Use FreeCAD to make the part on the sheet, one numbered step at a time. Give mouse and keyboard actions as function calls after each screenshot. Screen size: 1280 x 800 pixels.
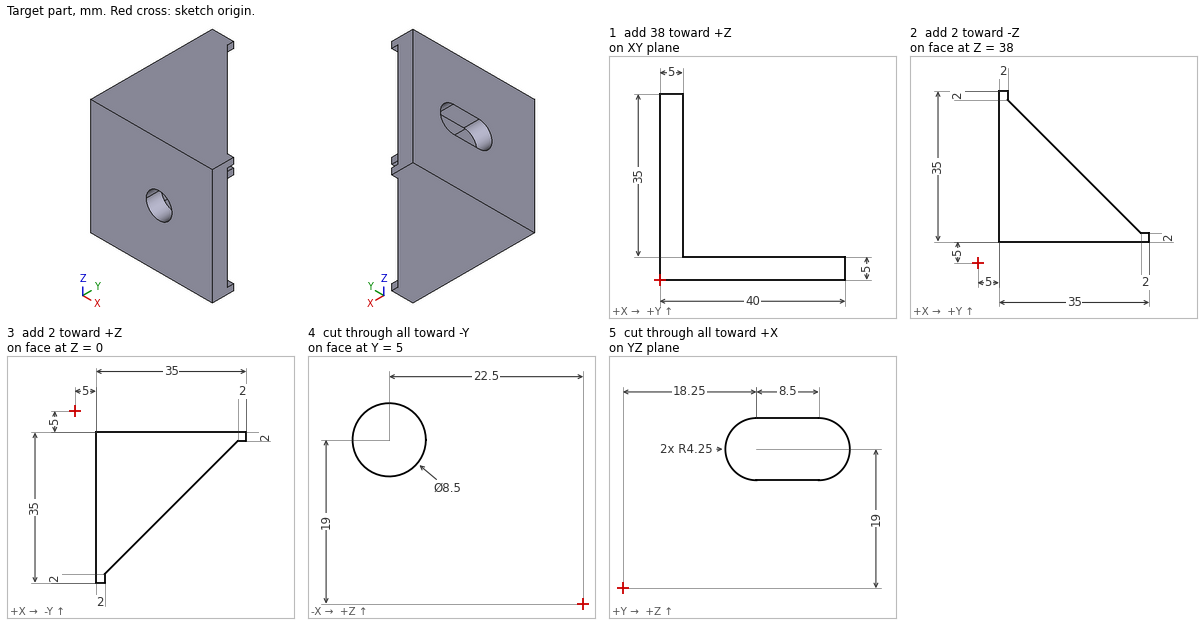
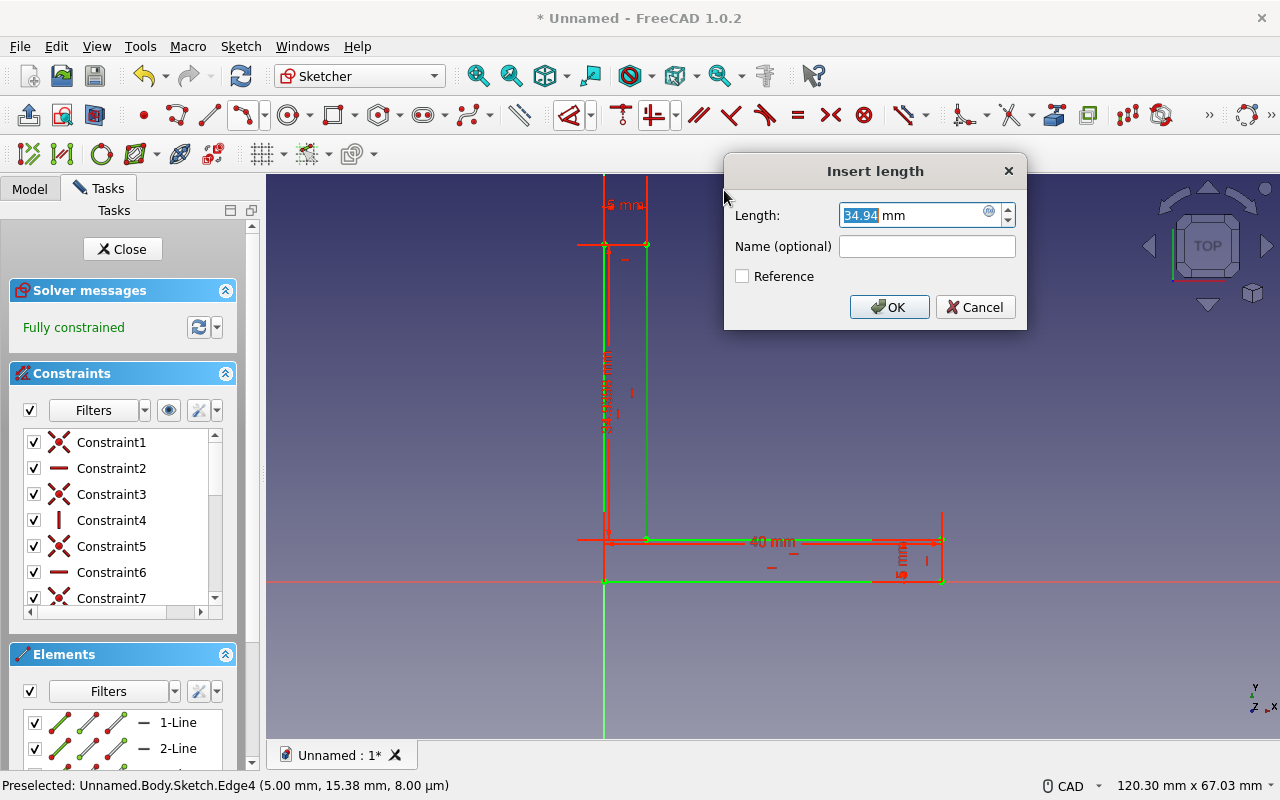
text(35)
key(Return)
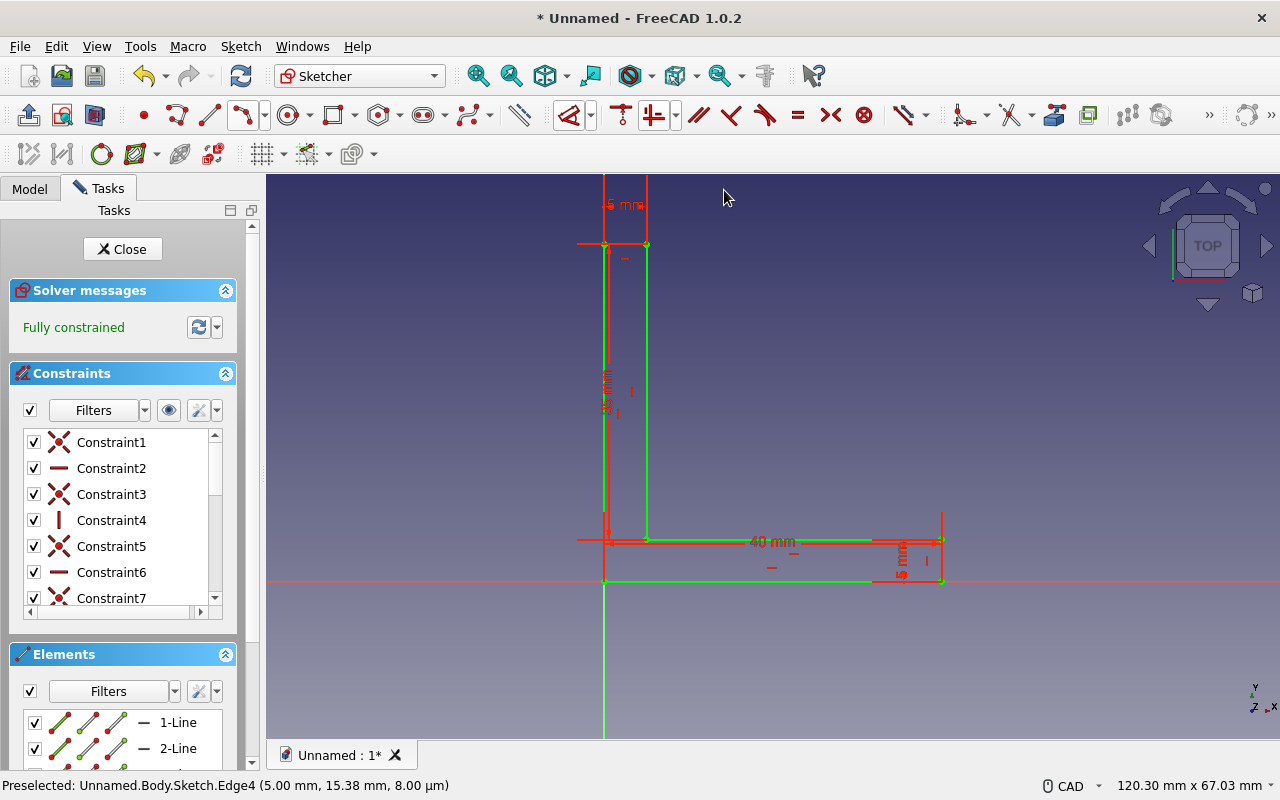
click(123, 249)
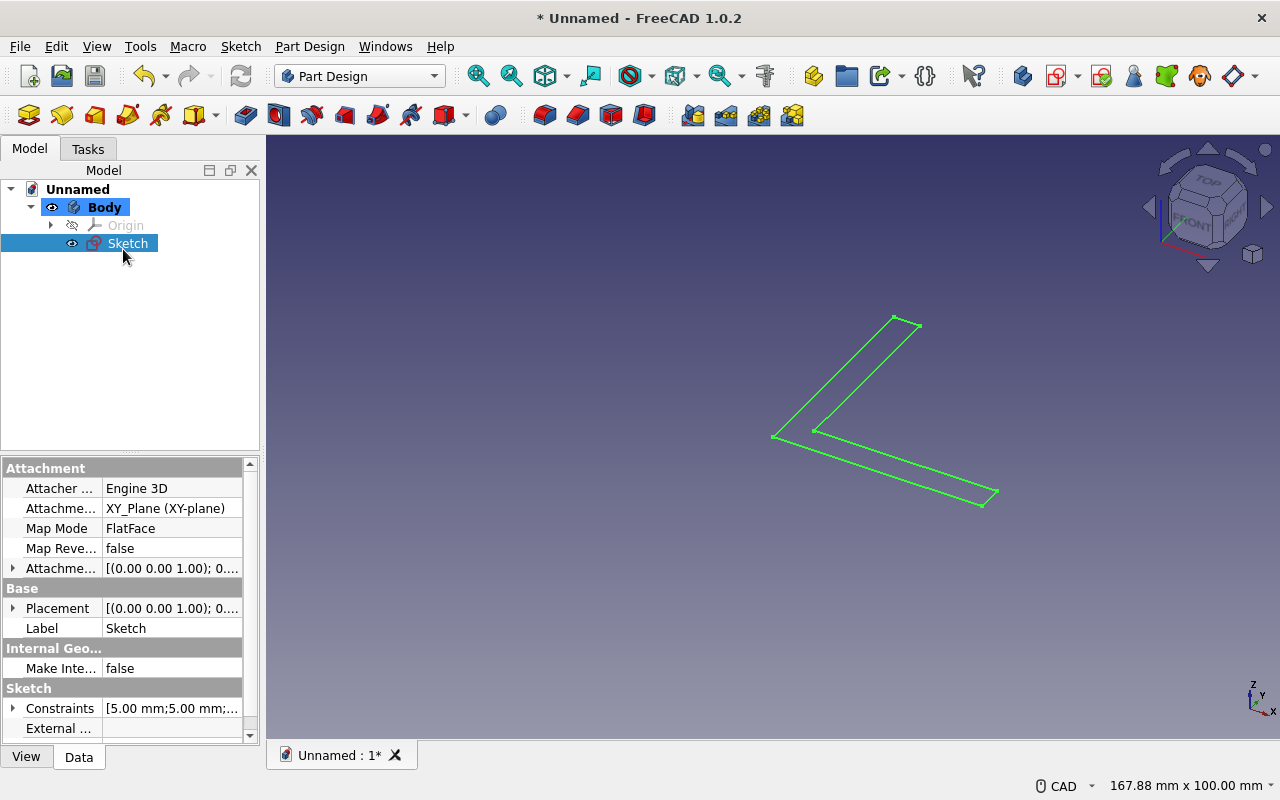
click(29, 116)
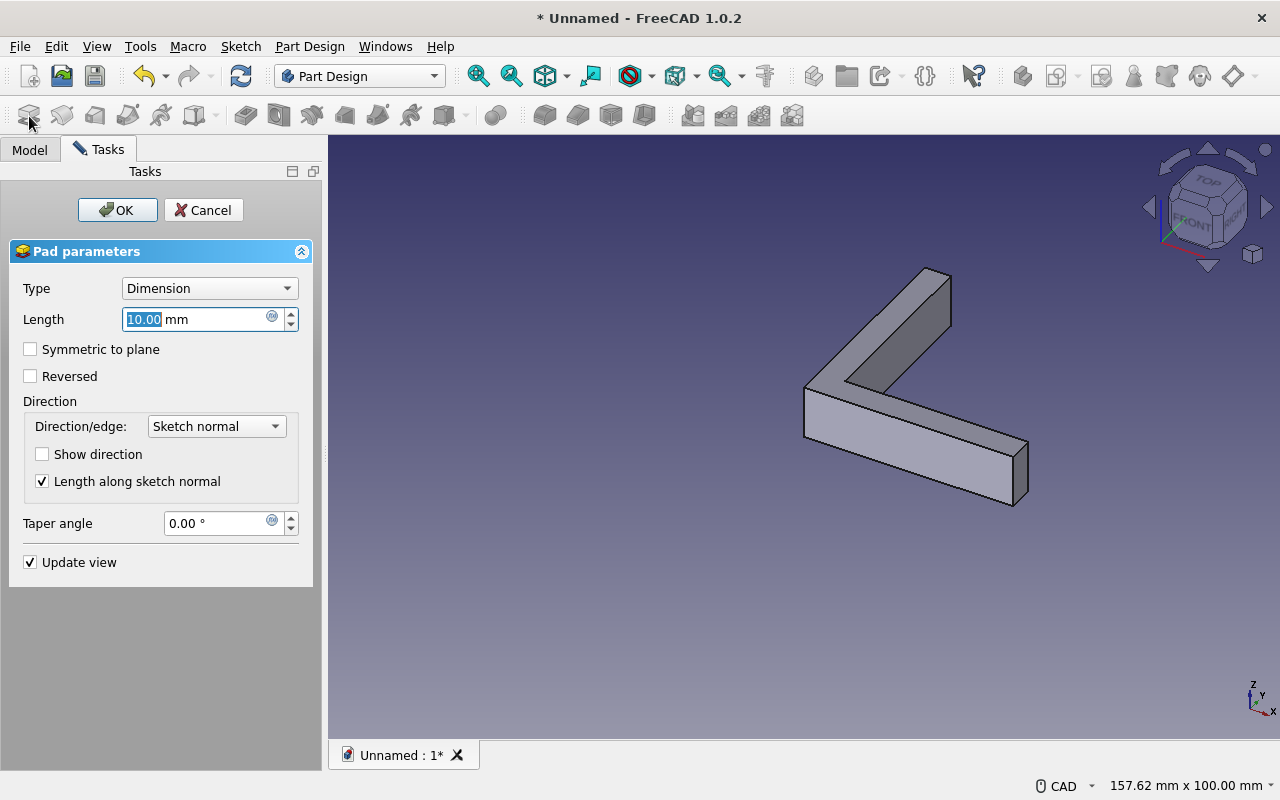
text(38)
key(Tab)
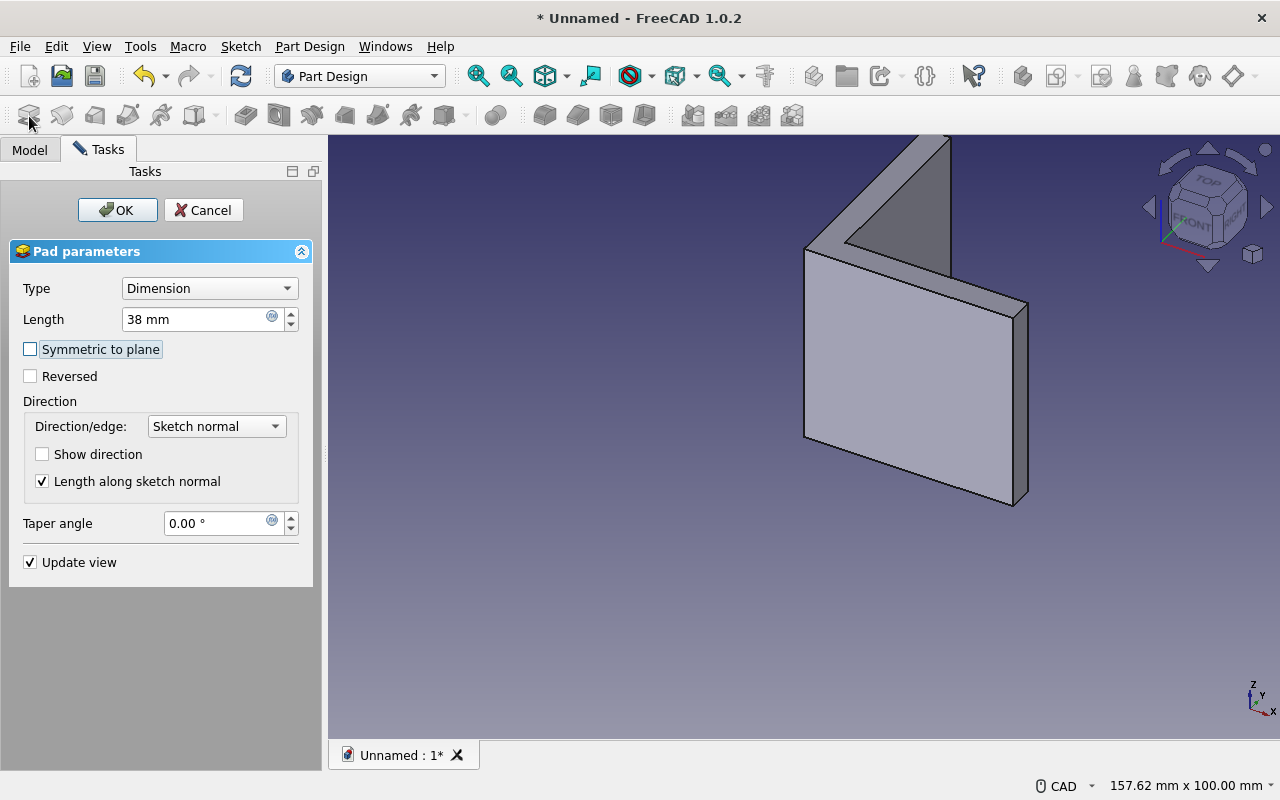
click(118, 210)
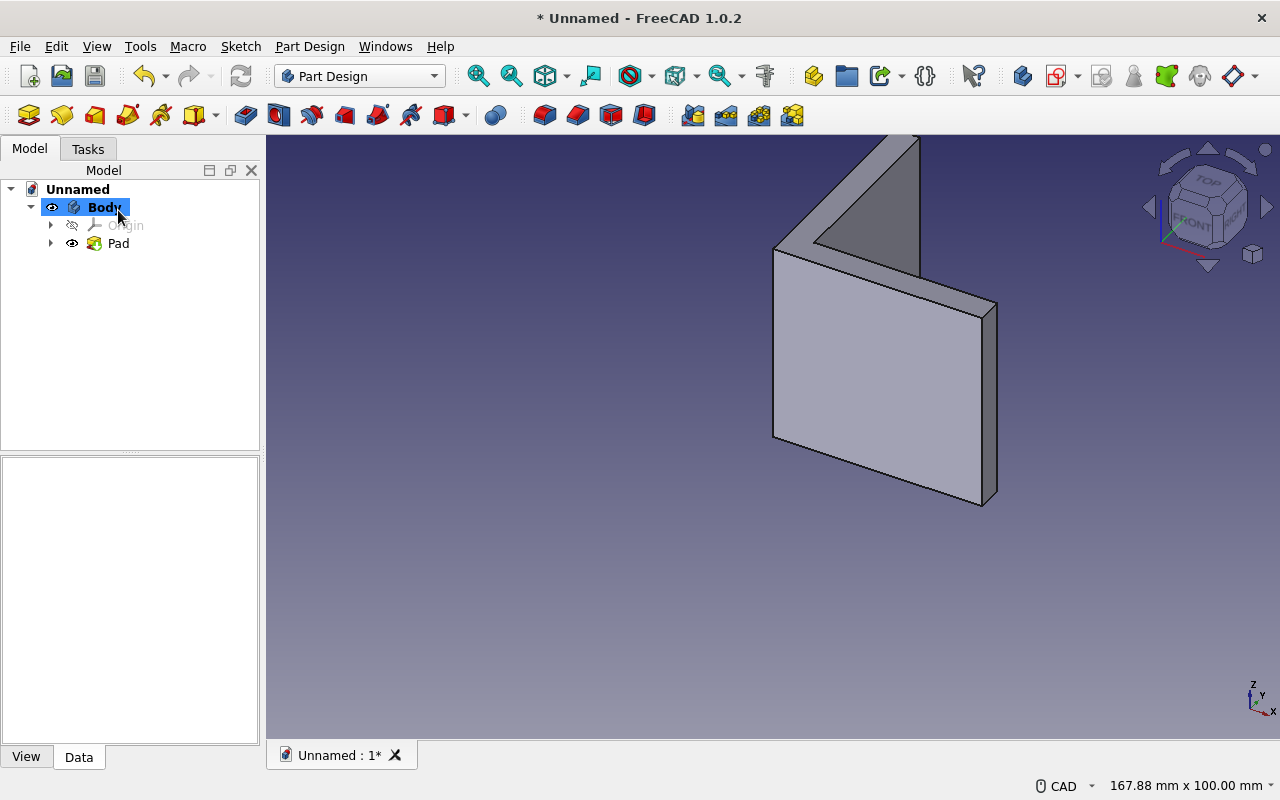
click(479, 76)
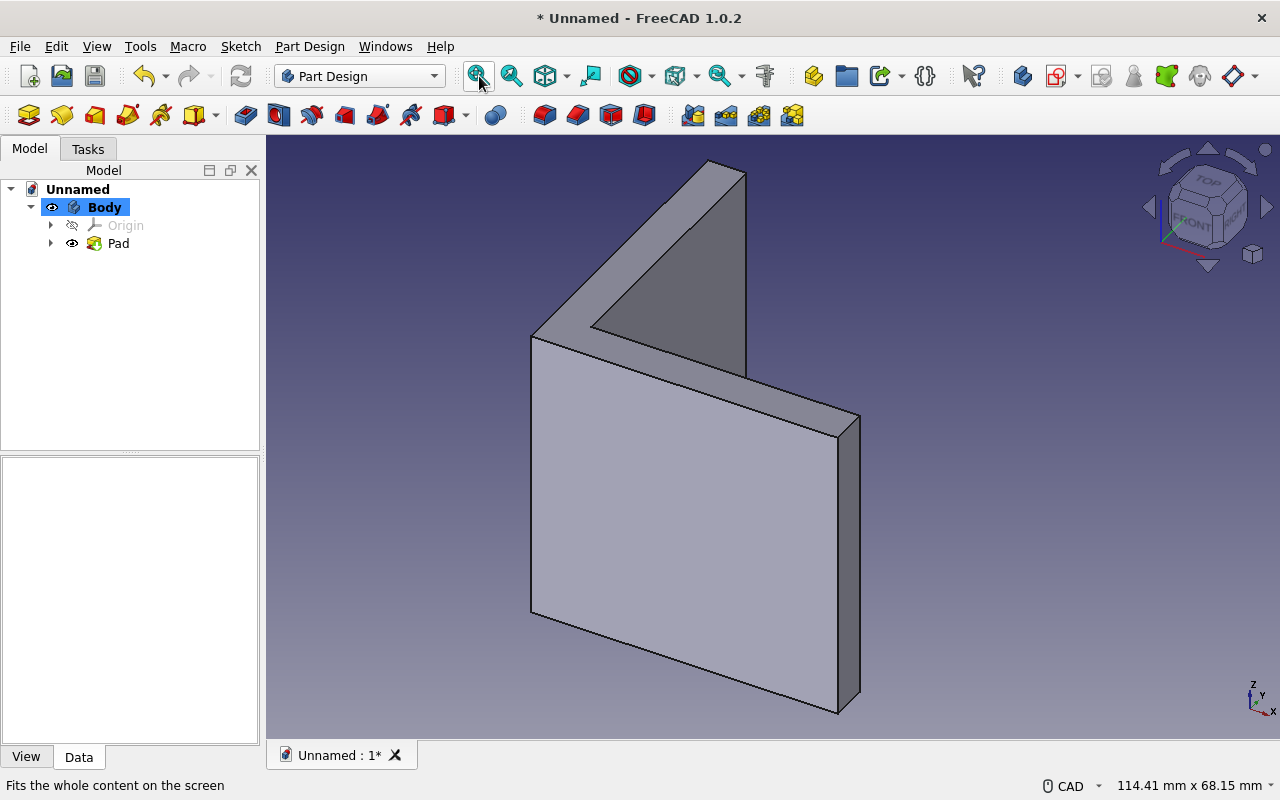
click(565, 330)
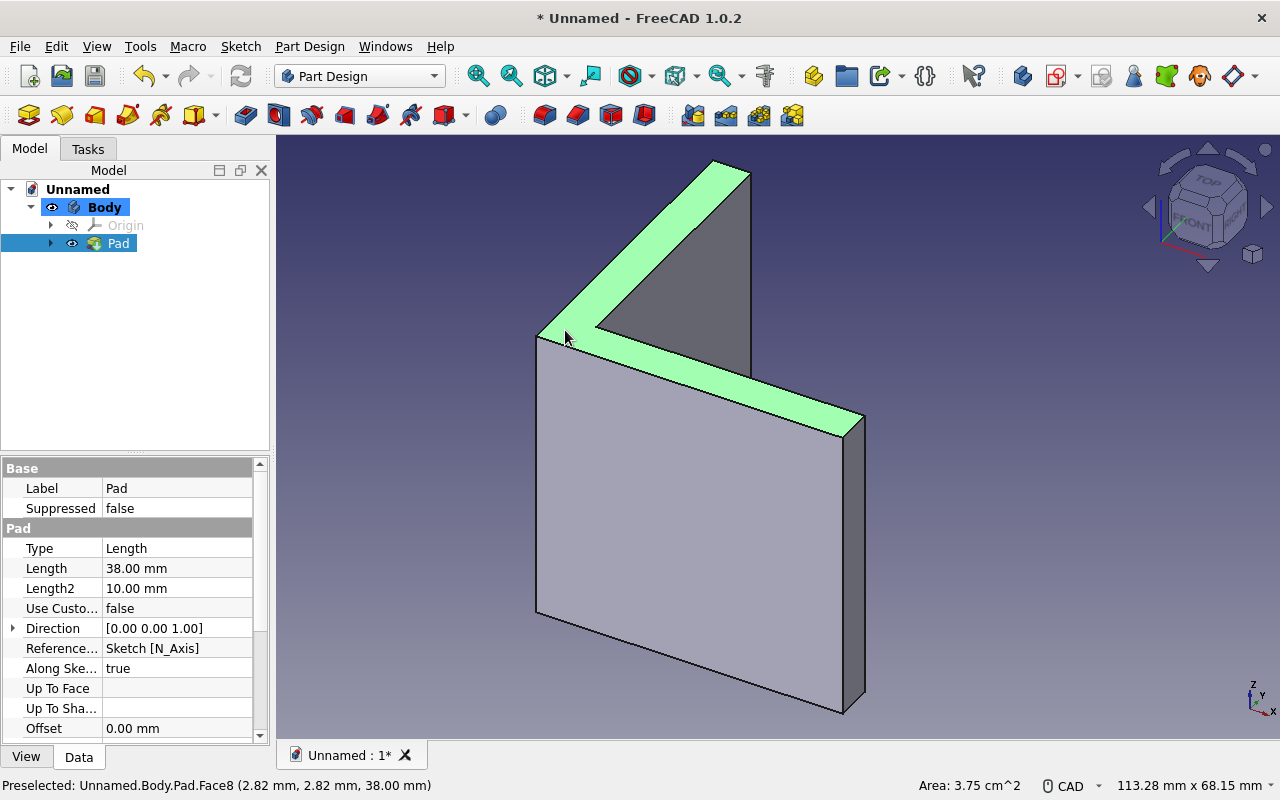
click(1056, 76)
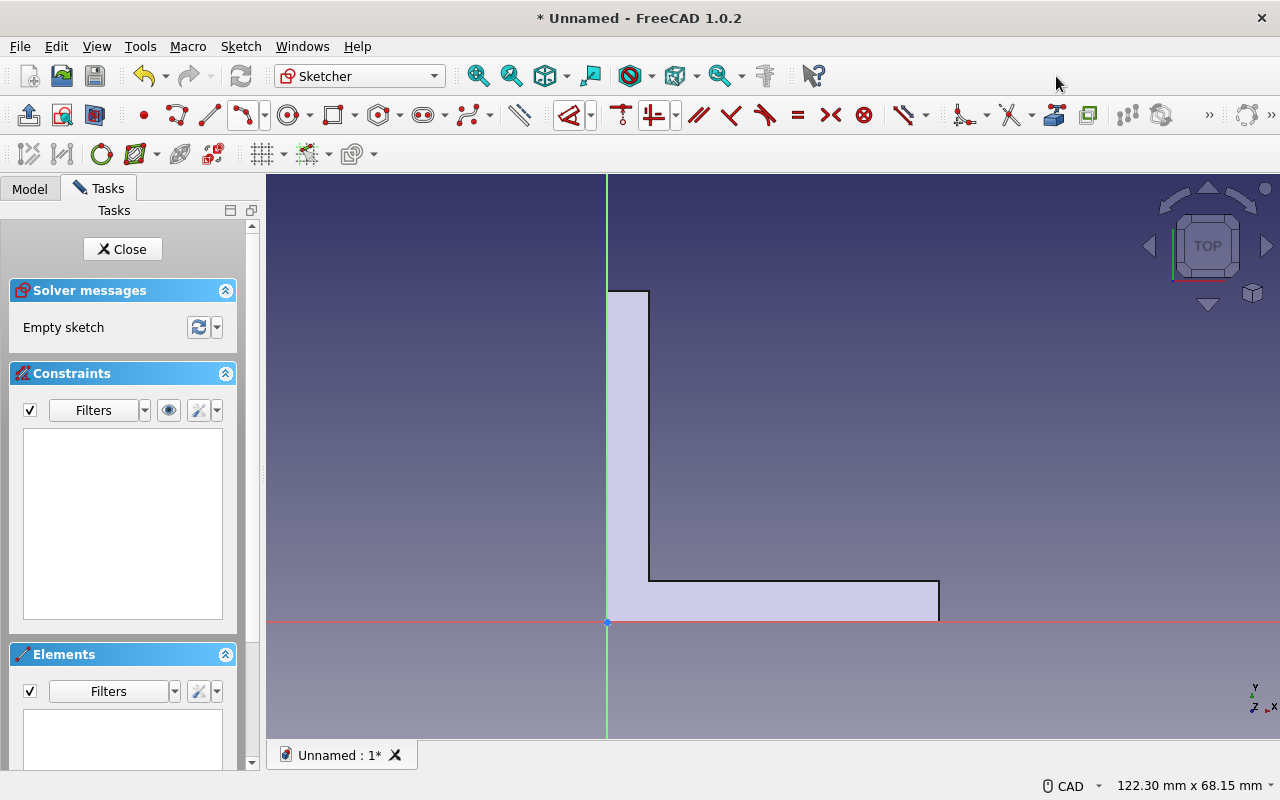
click(177, 116)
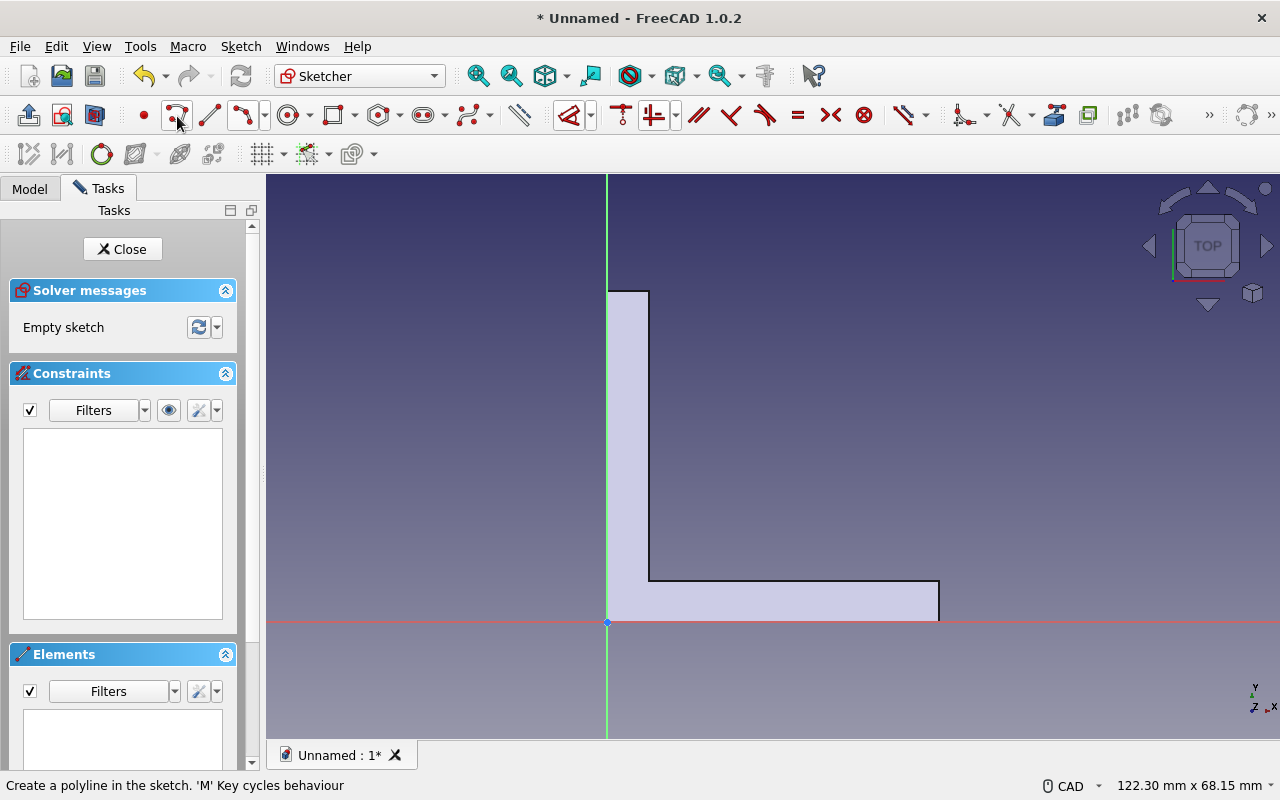
click(649, 581)
click(939, 581)
click(939, 564)
click(922, 564)
click(665, 307)
click(665, 291)
click(649, 291)
click(649, 582)
key(Escape)
key(Escape)